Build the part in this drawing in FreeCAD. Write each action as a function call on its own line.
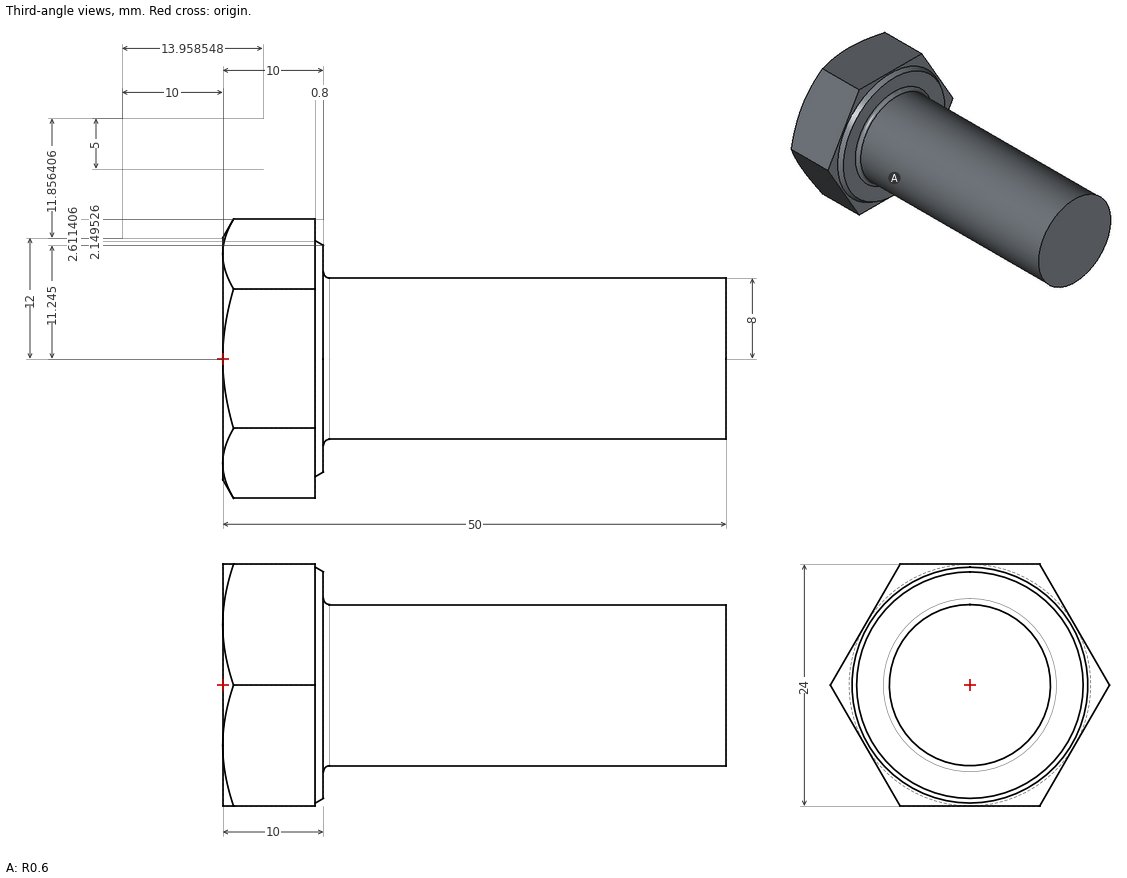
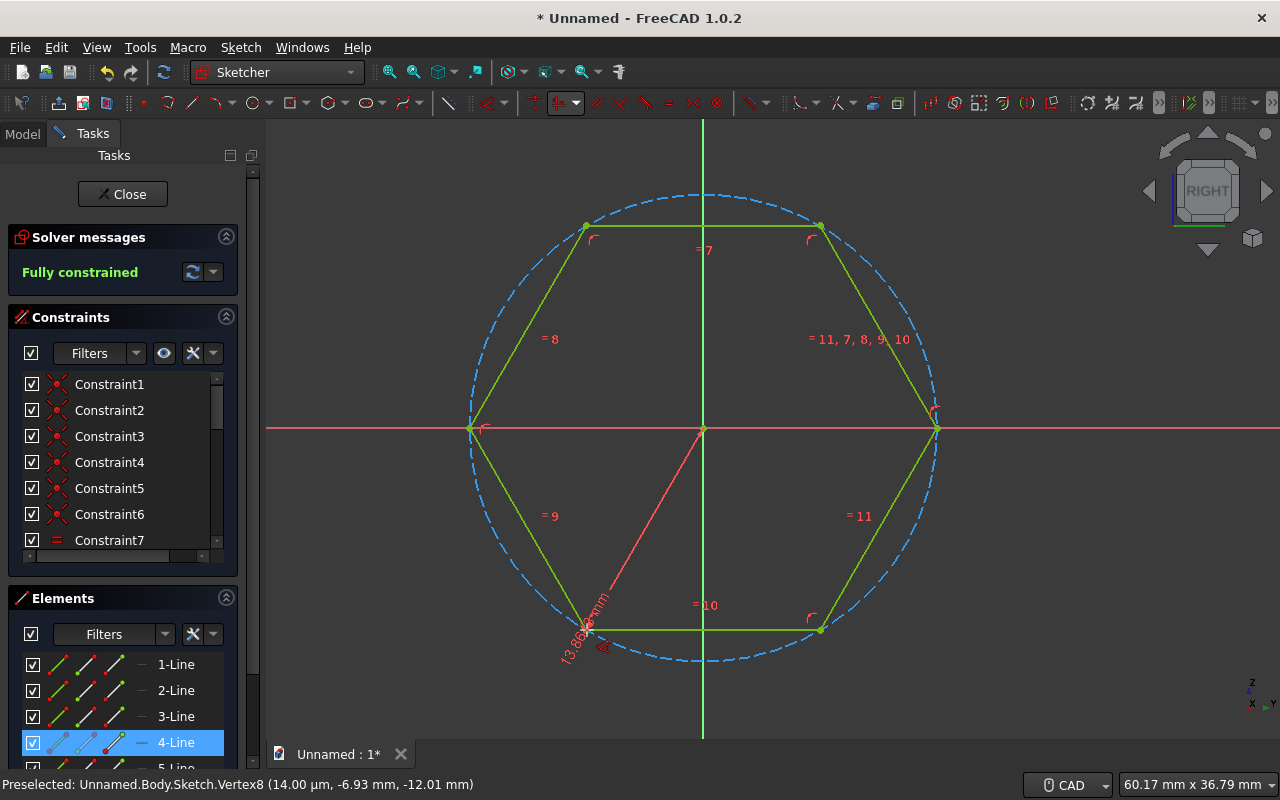
click(820, 226)
click(553, 335)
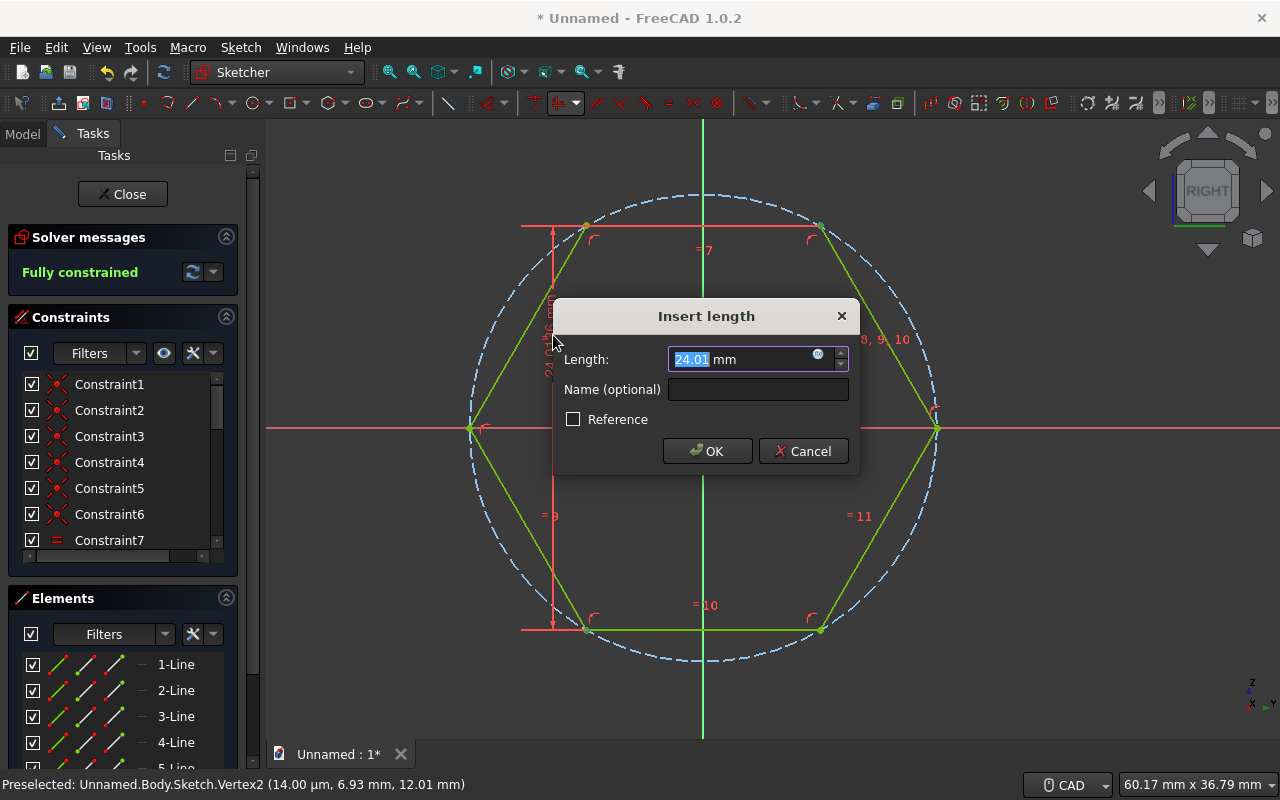
text(24)
key(Return)
key(Escape)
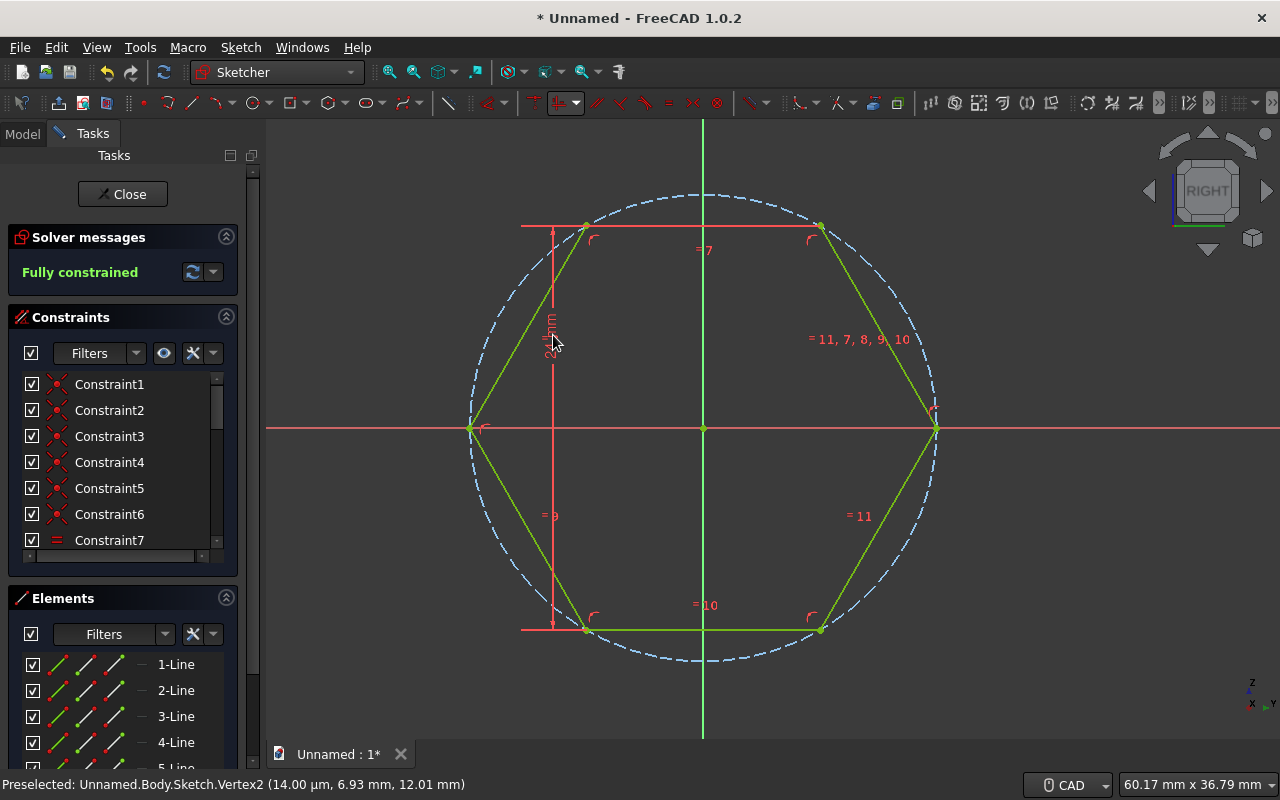
click(123, 194)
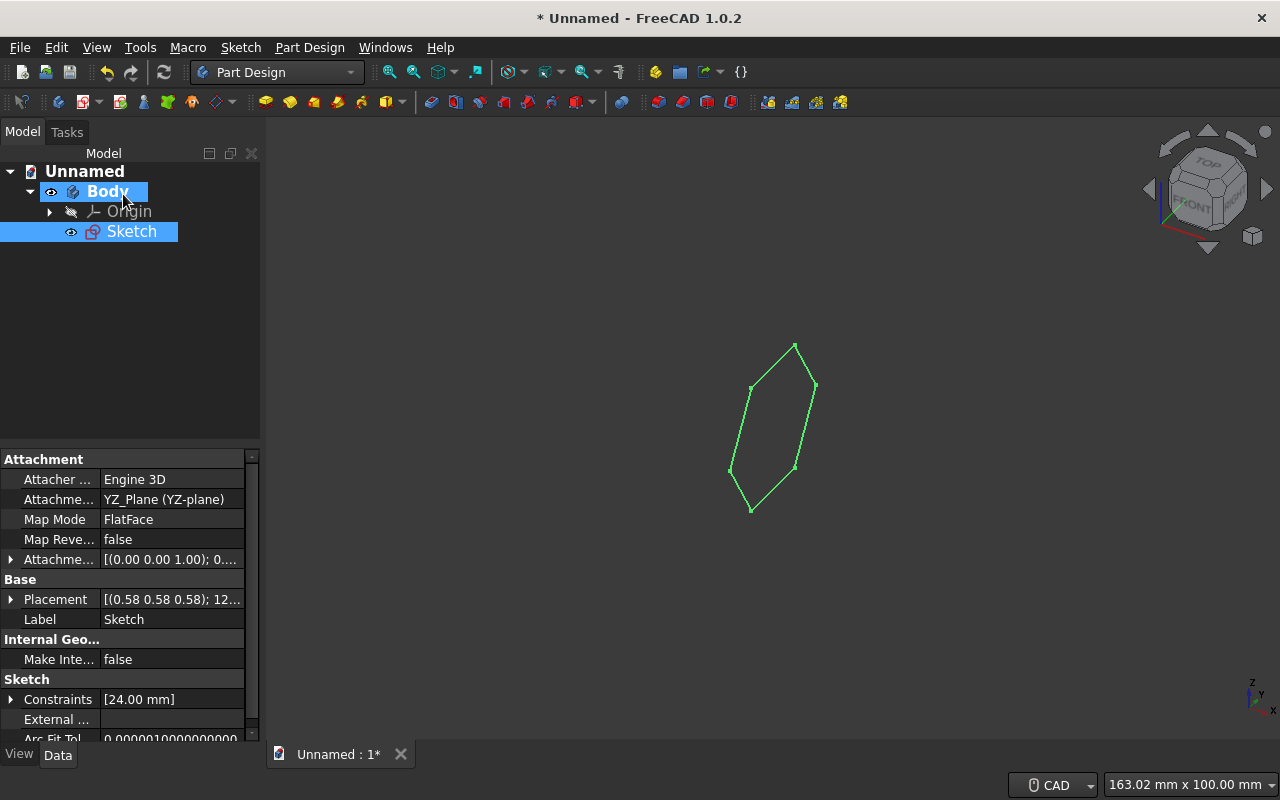
click(266, 102)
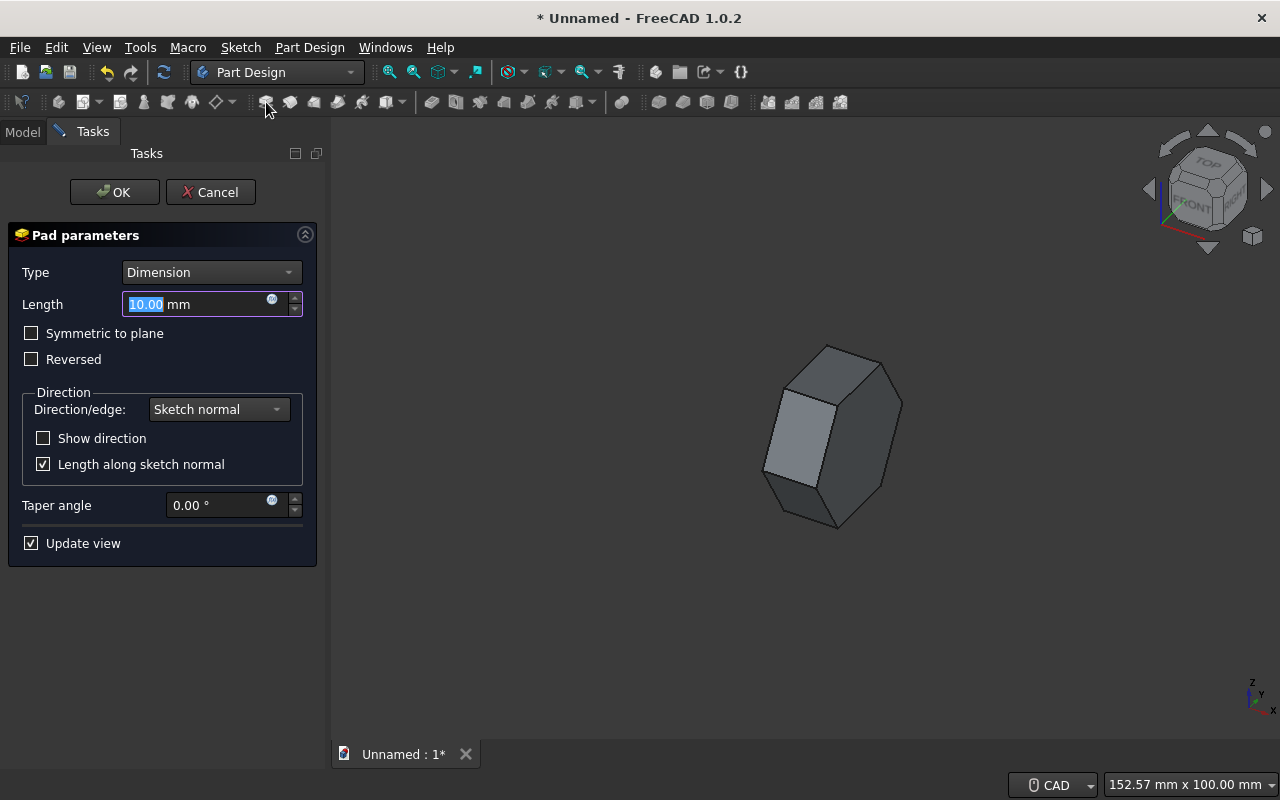
text(10)
key(Tab)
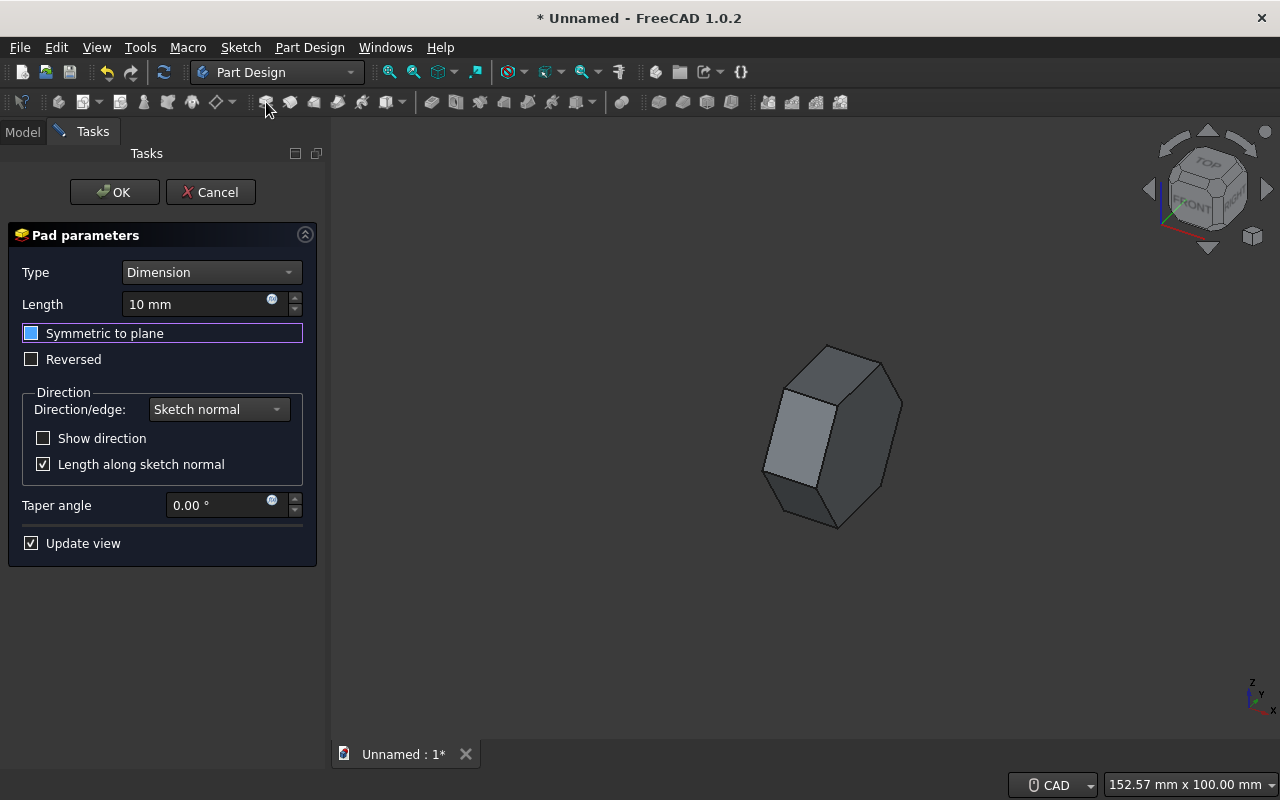
click(115, 192)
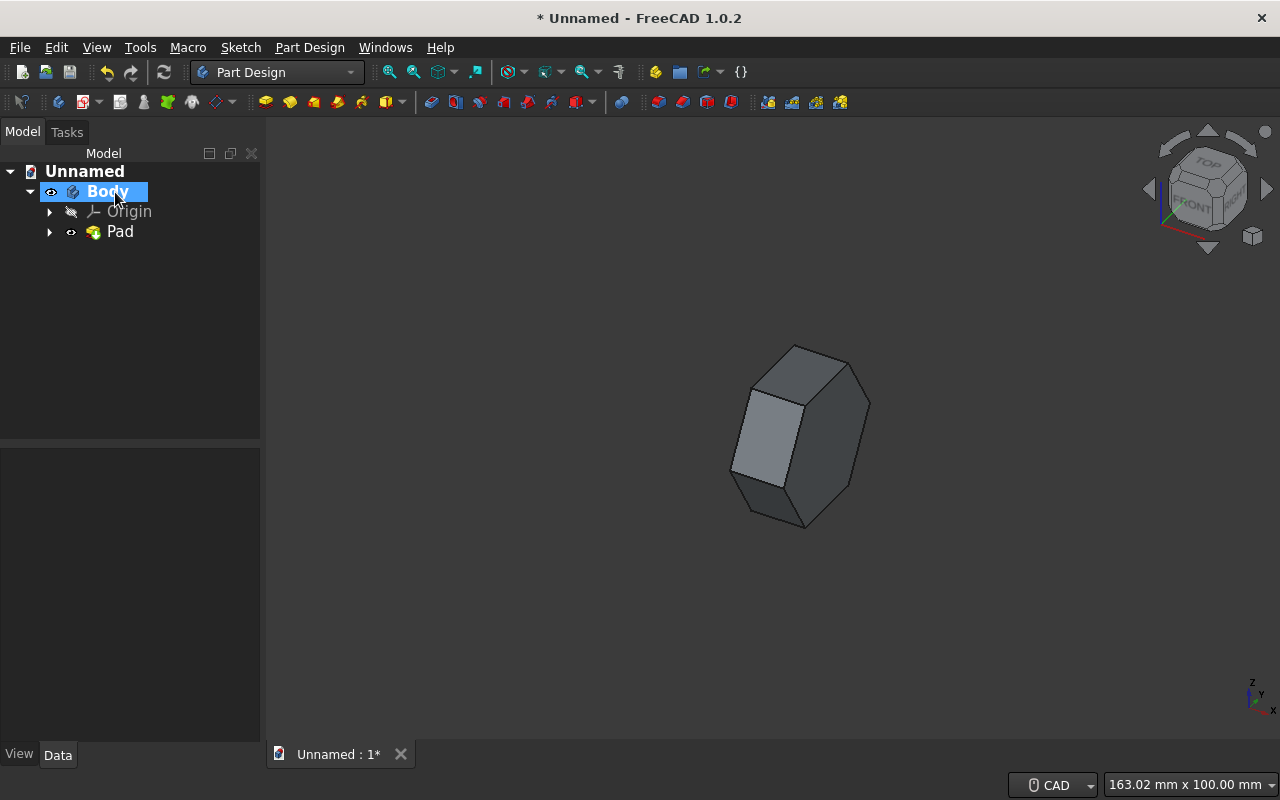
click(390, 72)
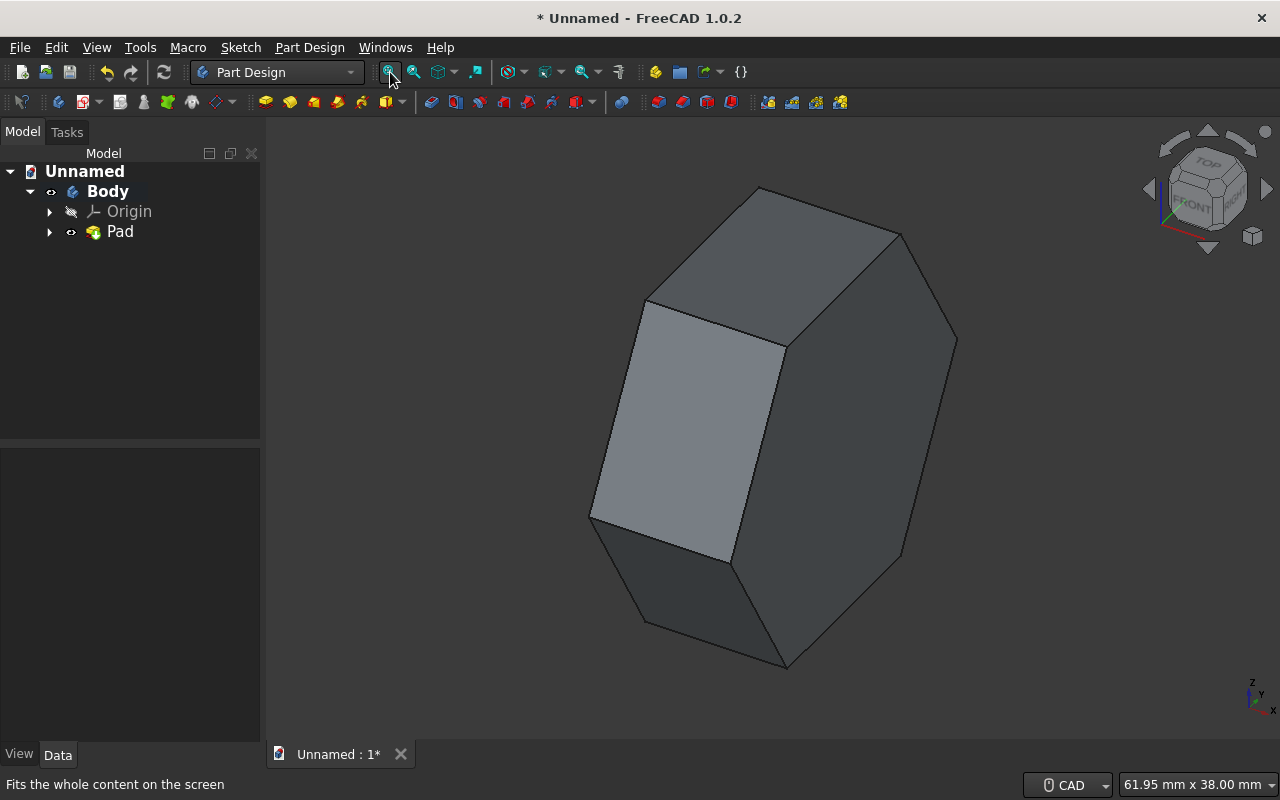
click(84, 102)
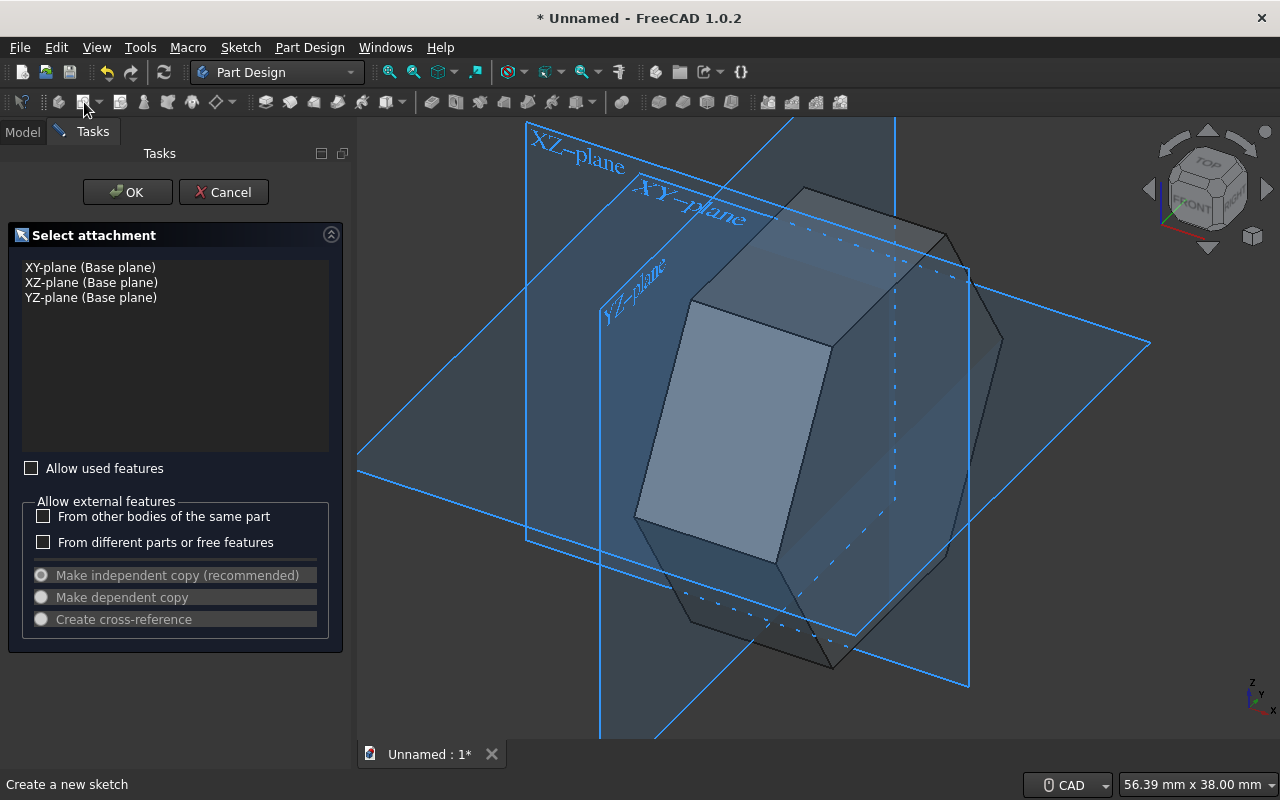
click(82, 268)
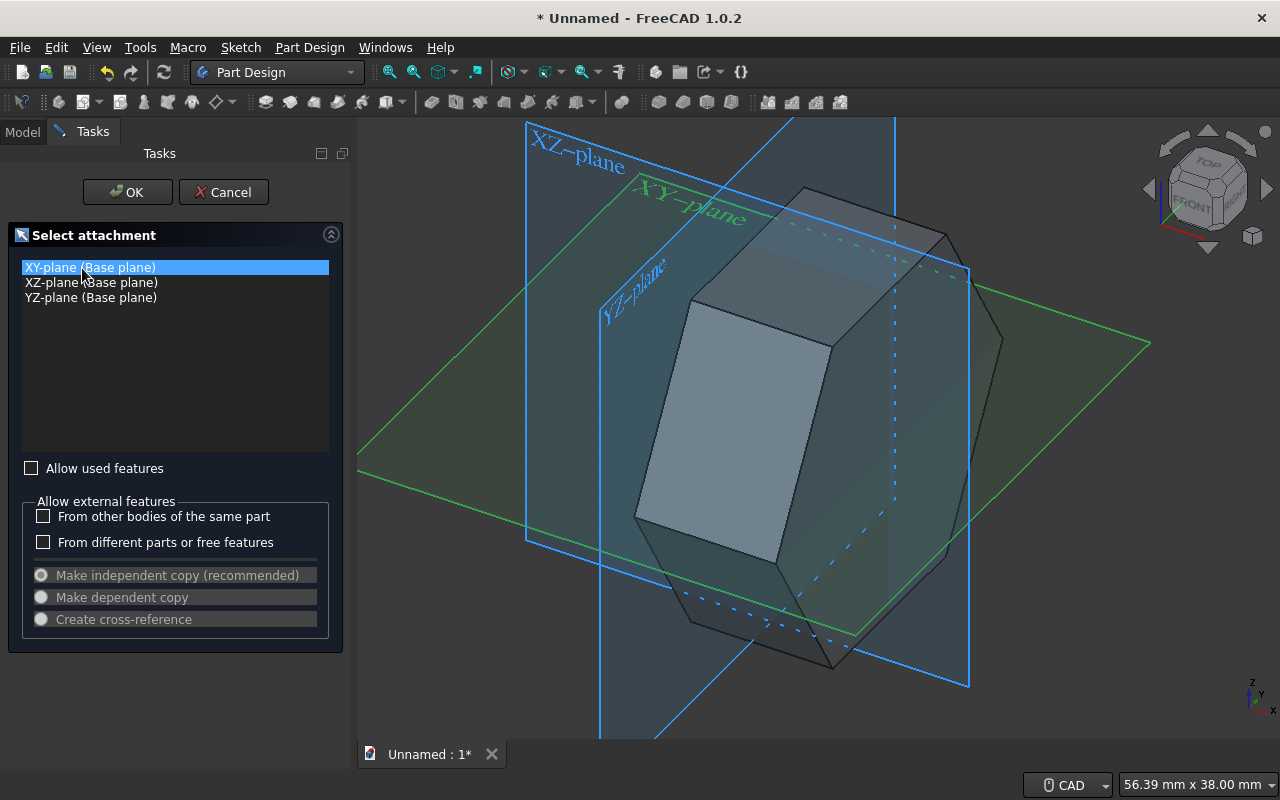
click(128, 192)